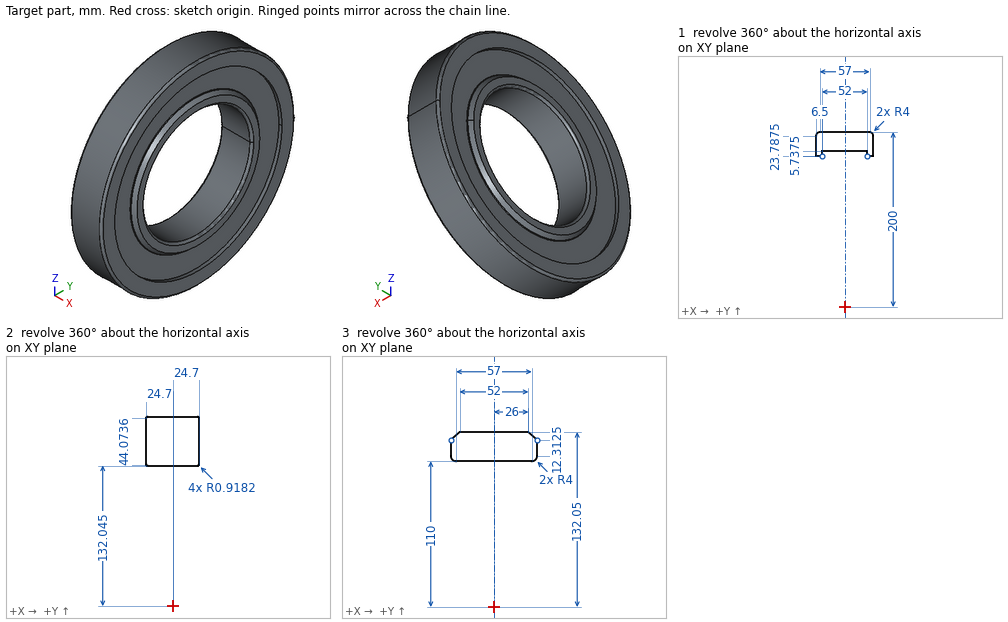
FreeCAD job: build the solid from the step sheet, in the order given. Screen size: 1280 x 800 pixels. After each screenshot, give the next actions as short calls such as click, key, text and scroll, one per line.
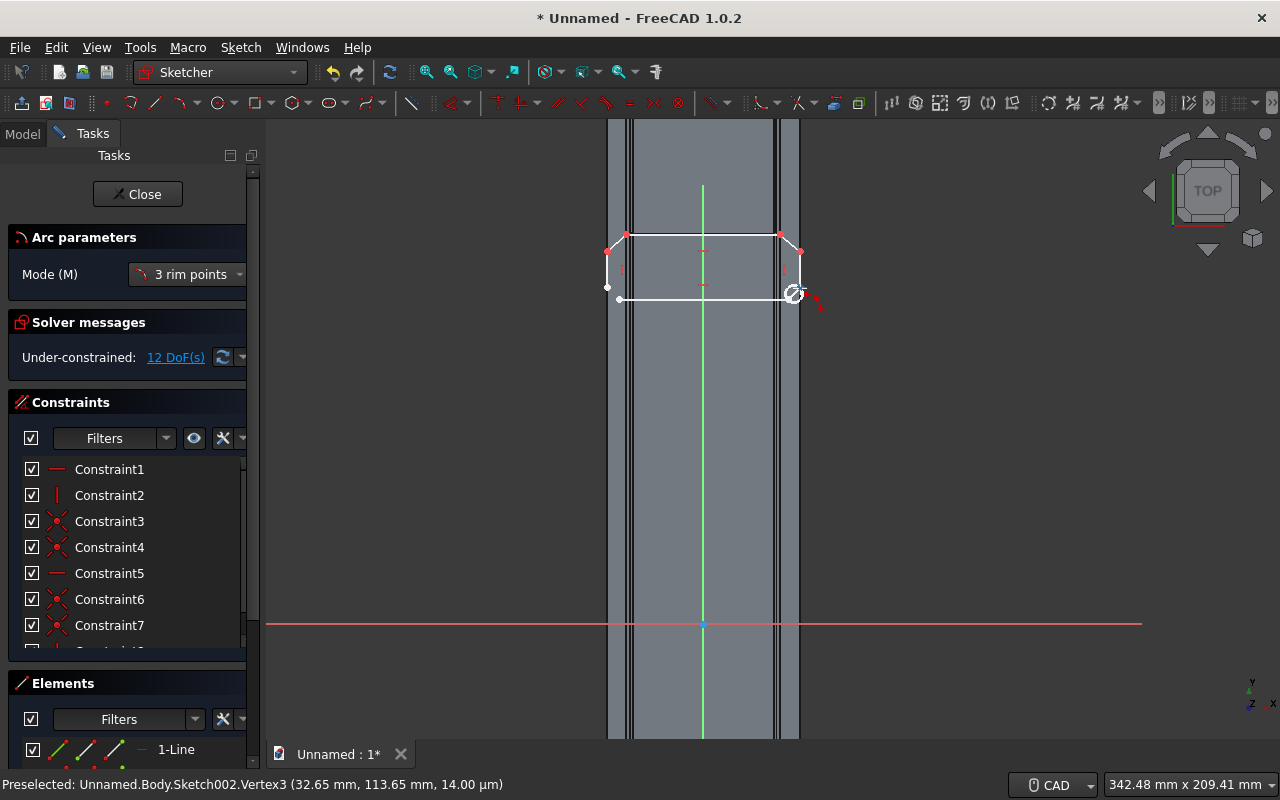
scroll(796, 295, up, 8)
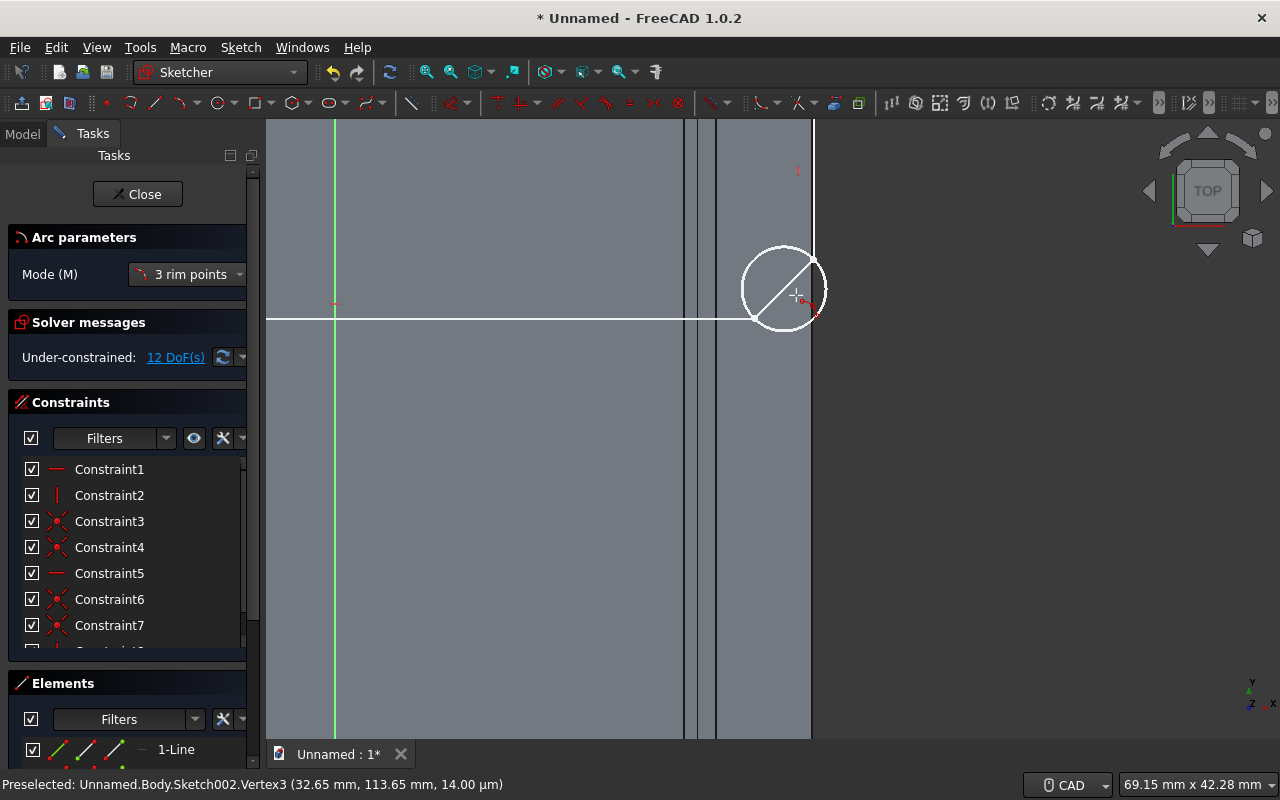
click(794, 296)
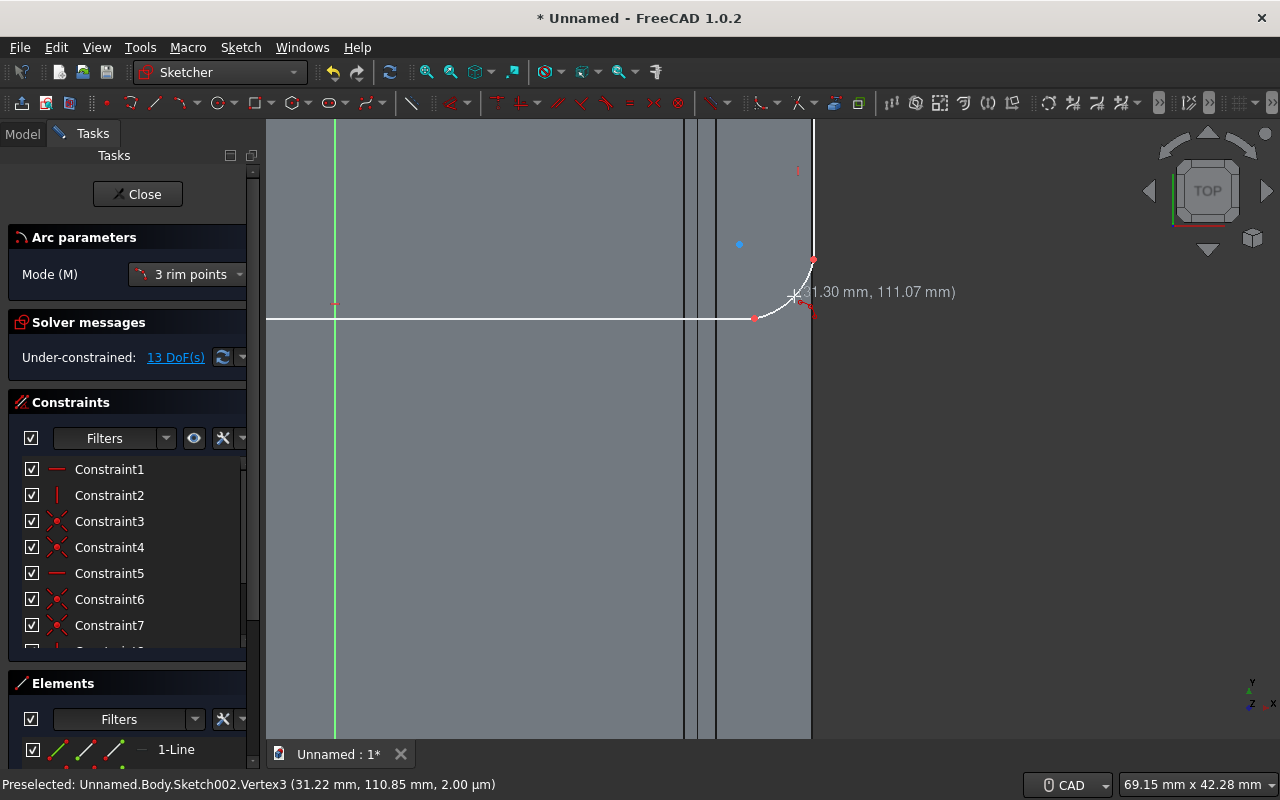
scroll(798, 295, down, 8)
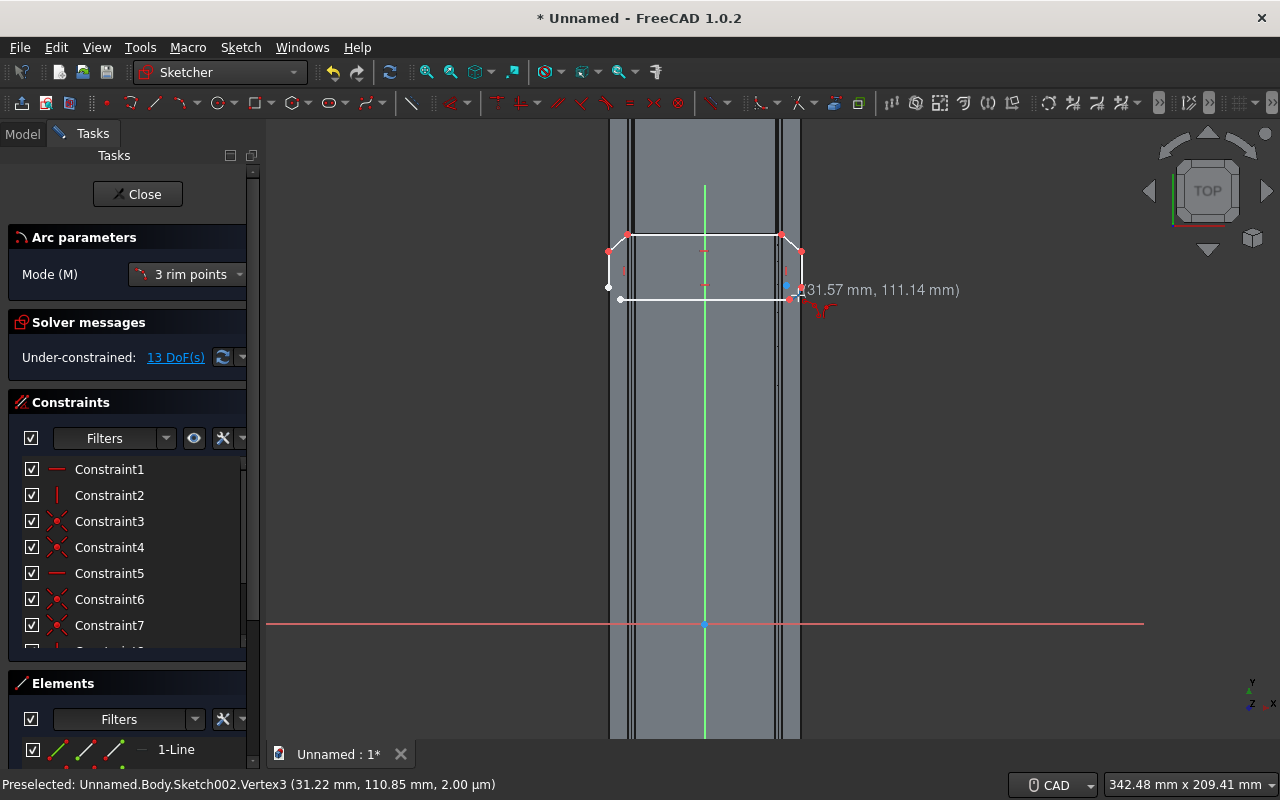
click(609, 288)
click(621, 300)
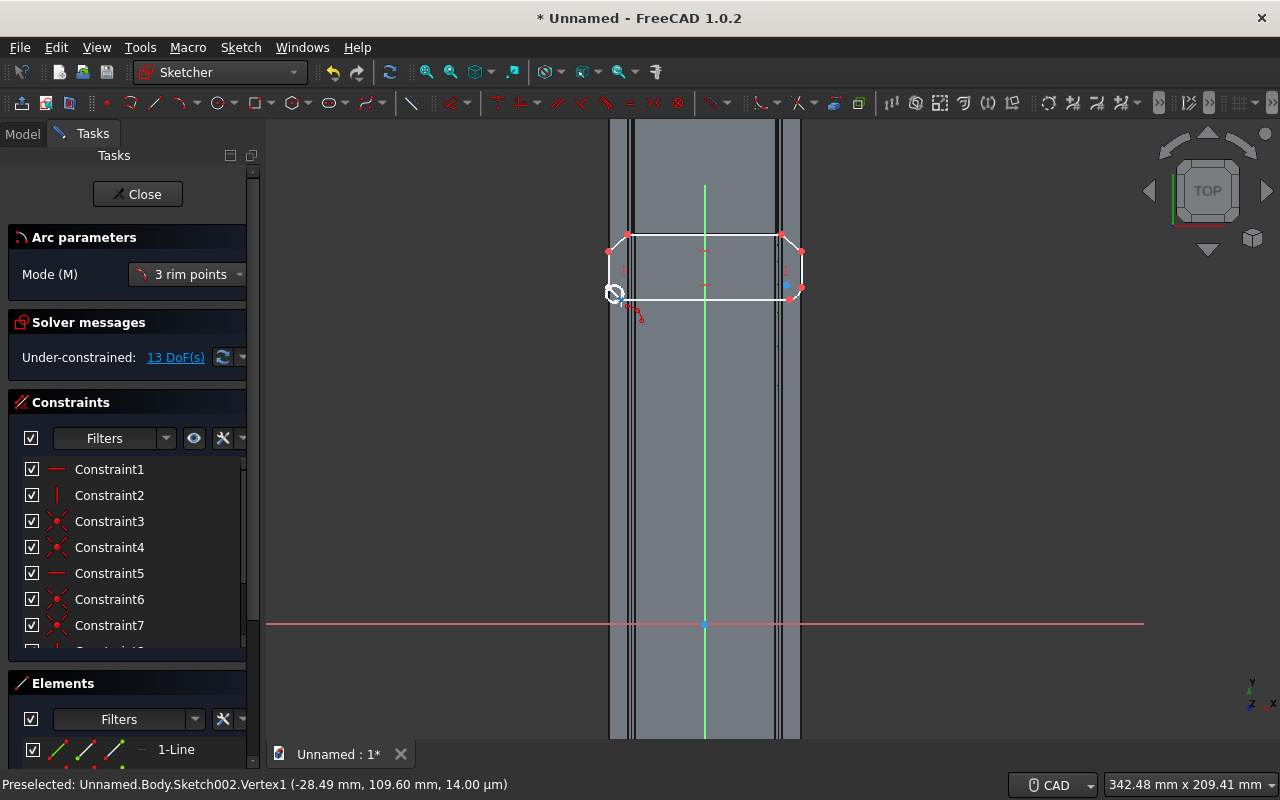
scroll(612, 295, up, 8)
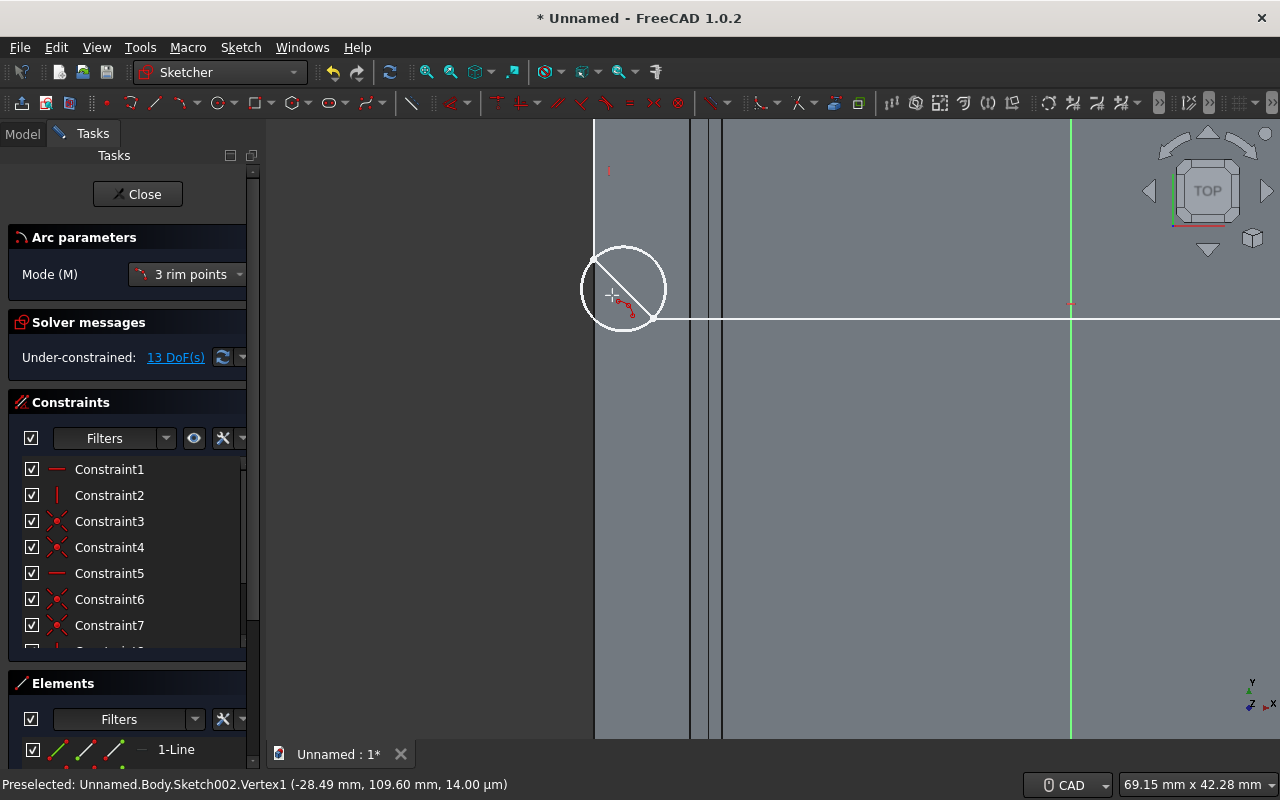
click(612, 296)
key(Escape)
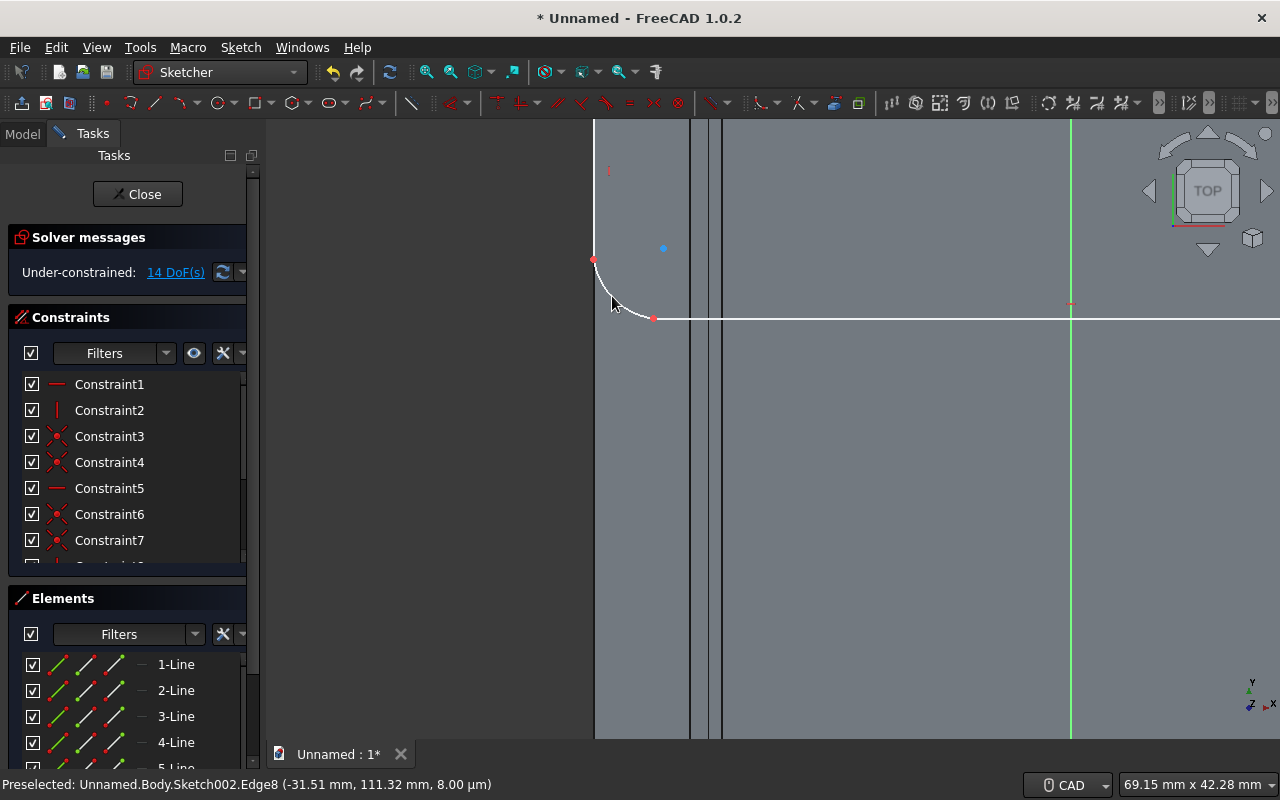
scroll(612, 295, down, 8)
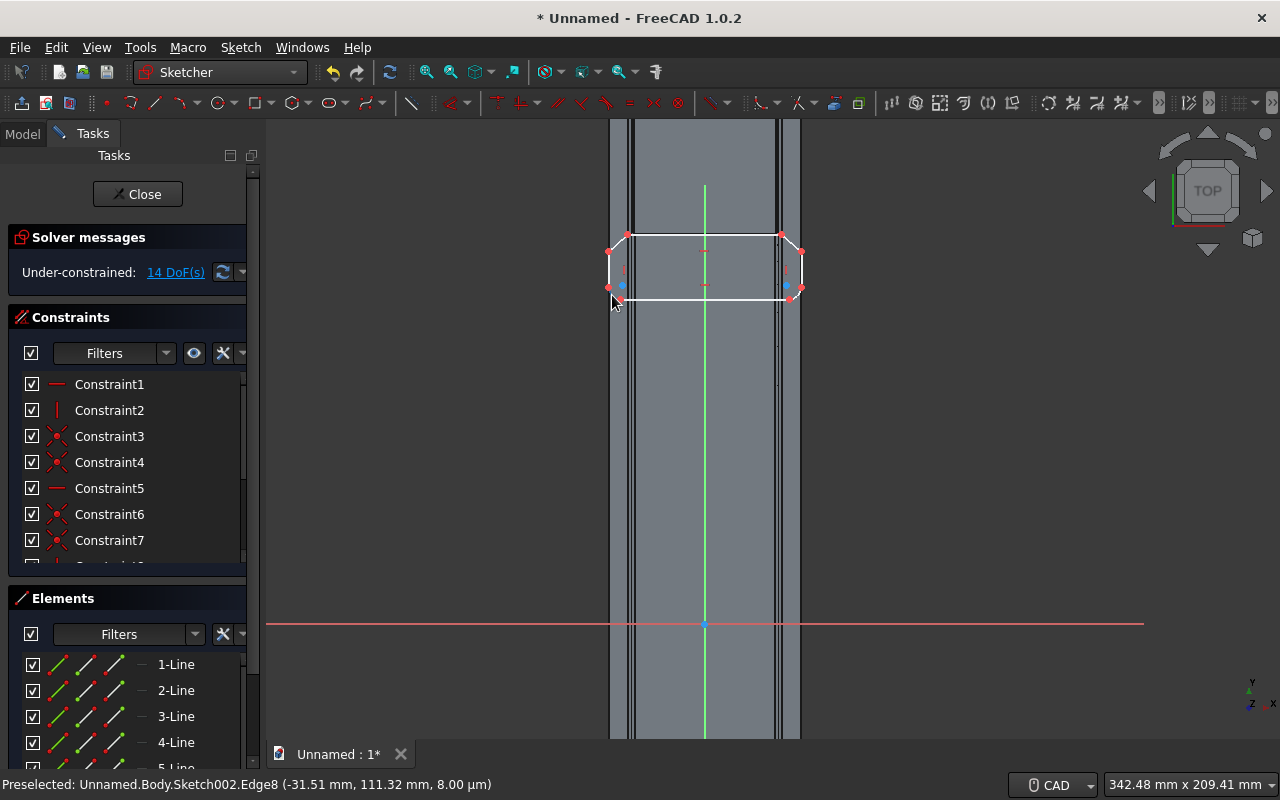
click(671, 300)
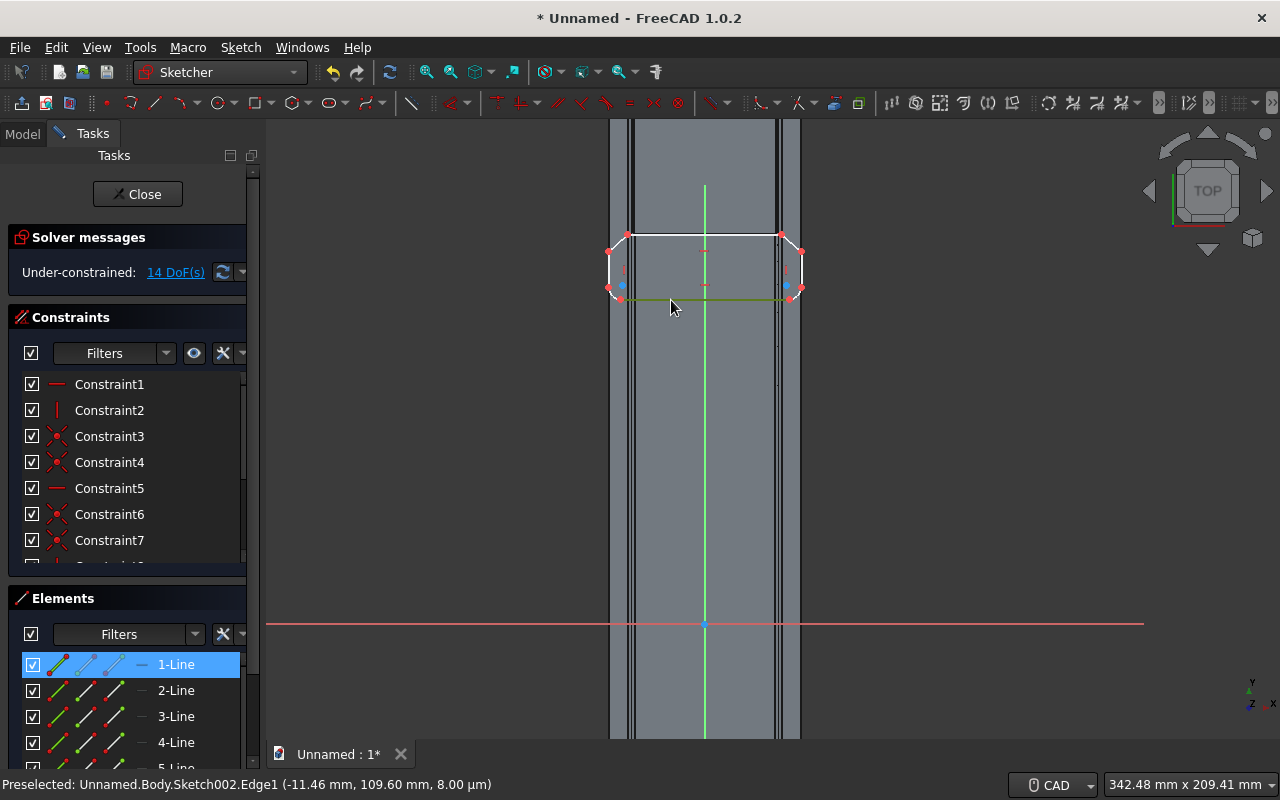
scroll(797, 296, up, 3)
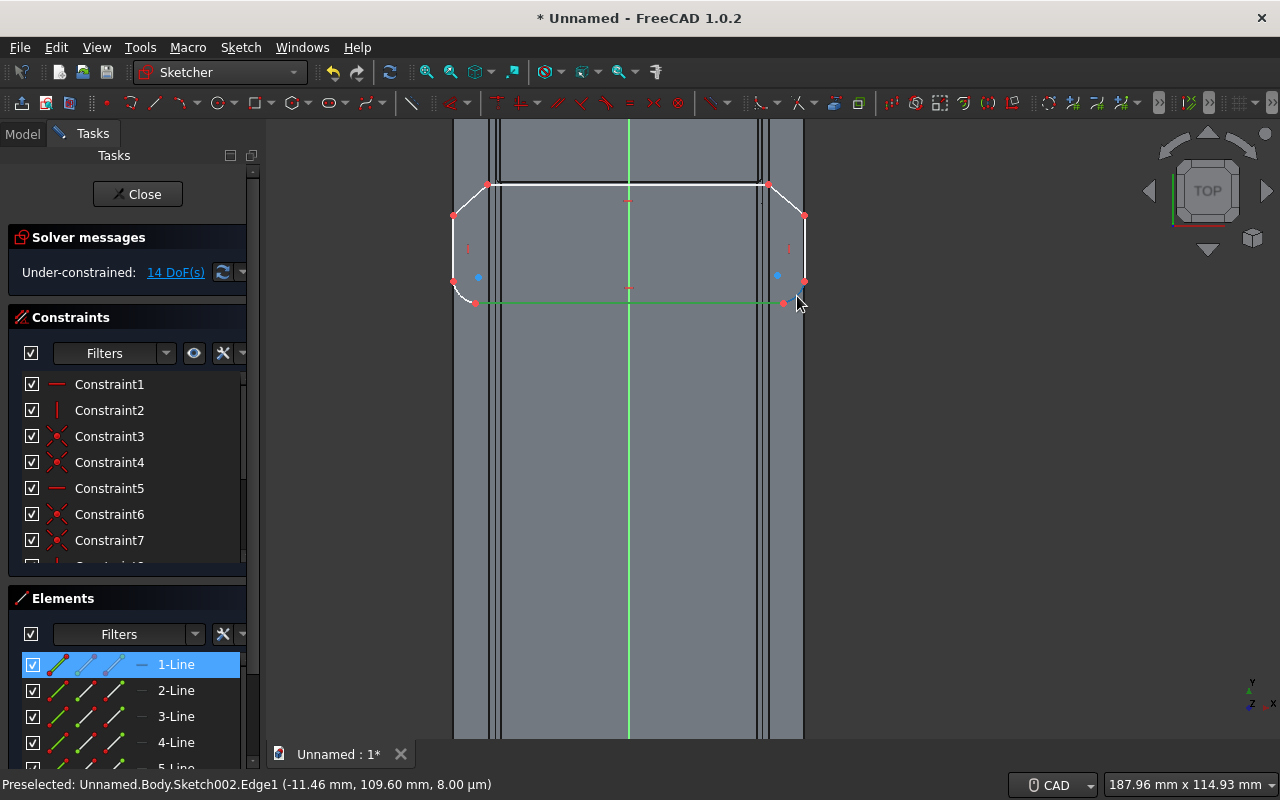
click(797, 295)